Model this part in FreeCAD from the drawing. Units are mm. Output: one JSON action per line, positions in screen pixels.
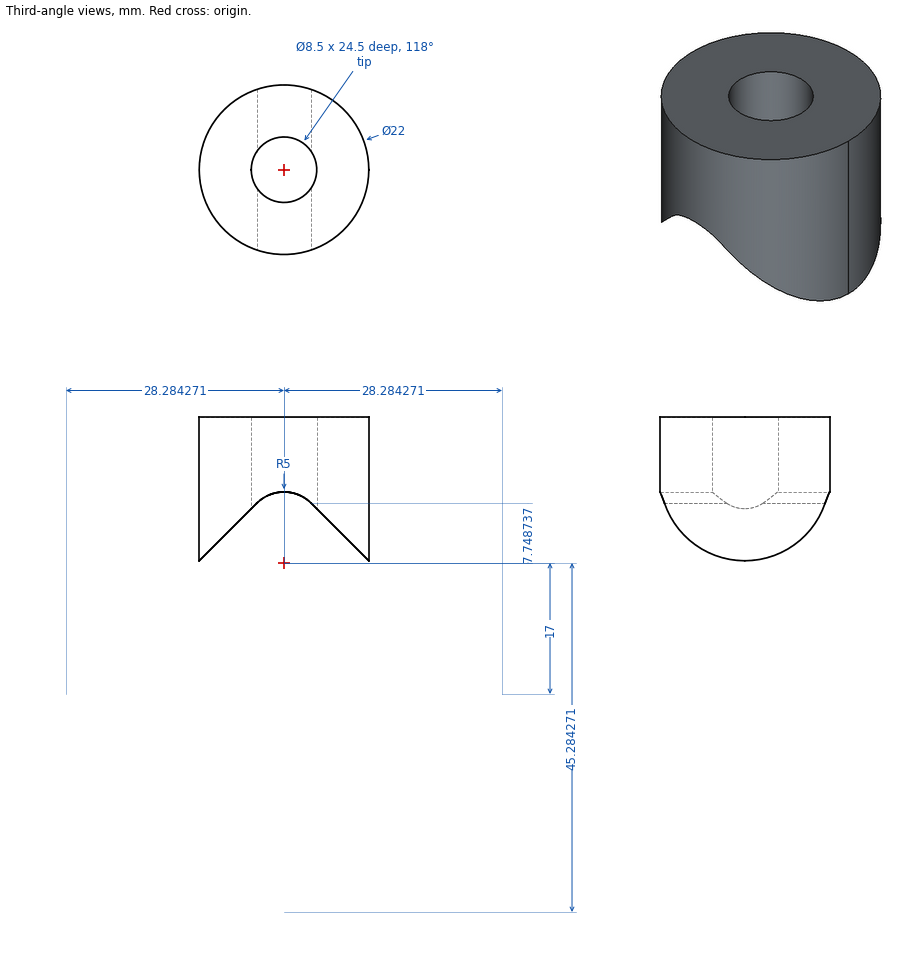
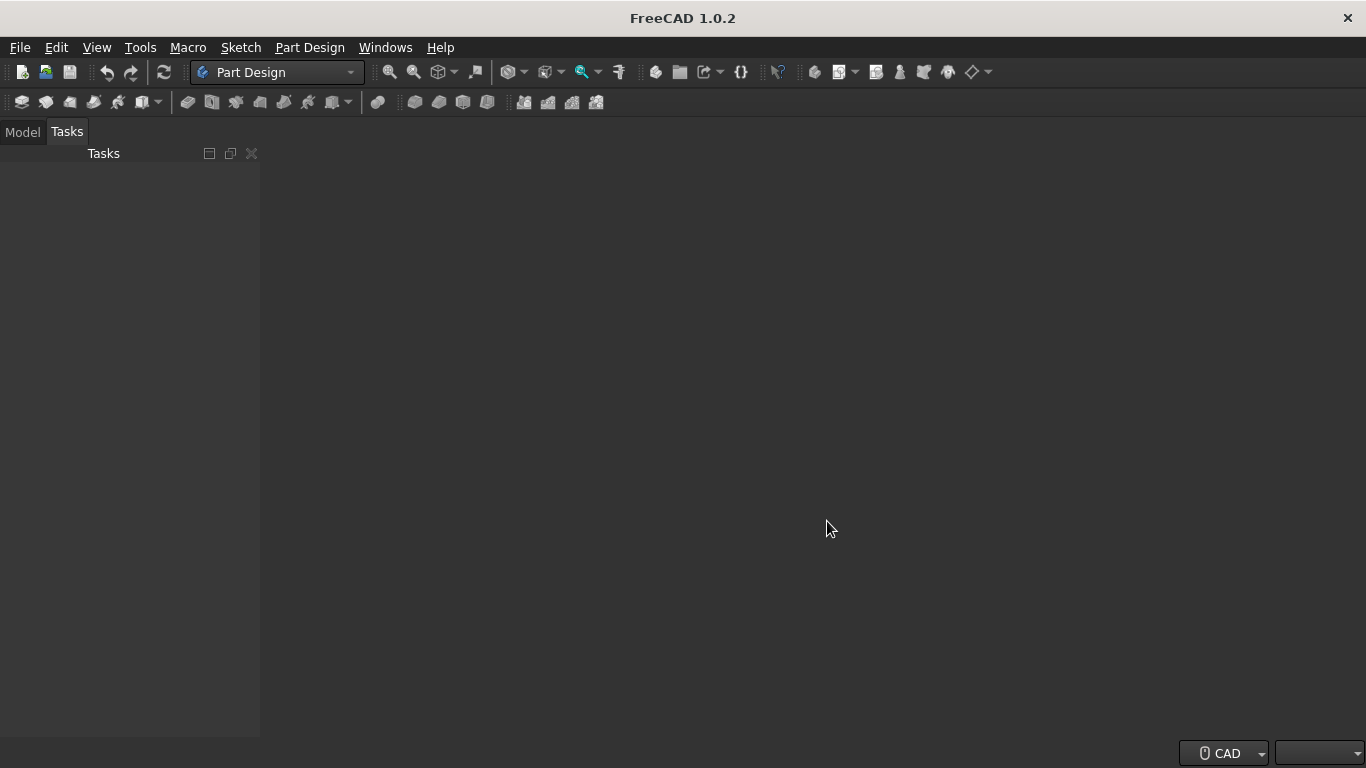
{"action": "key", "text": "ctrl+n"}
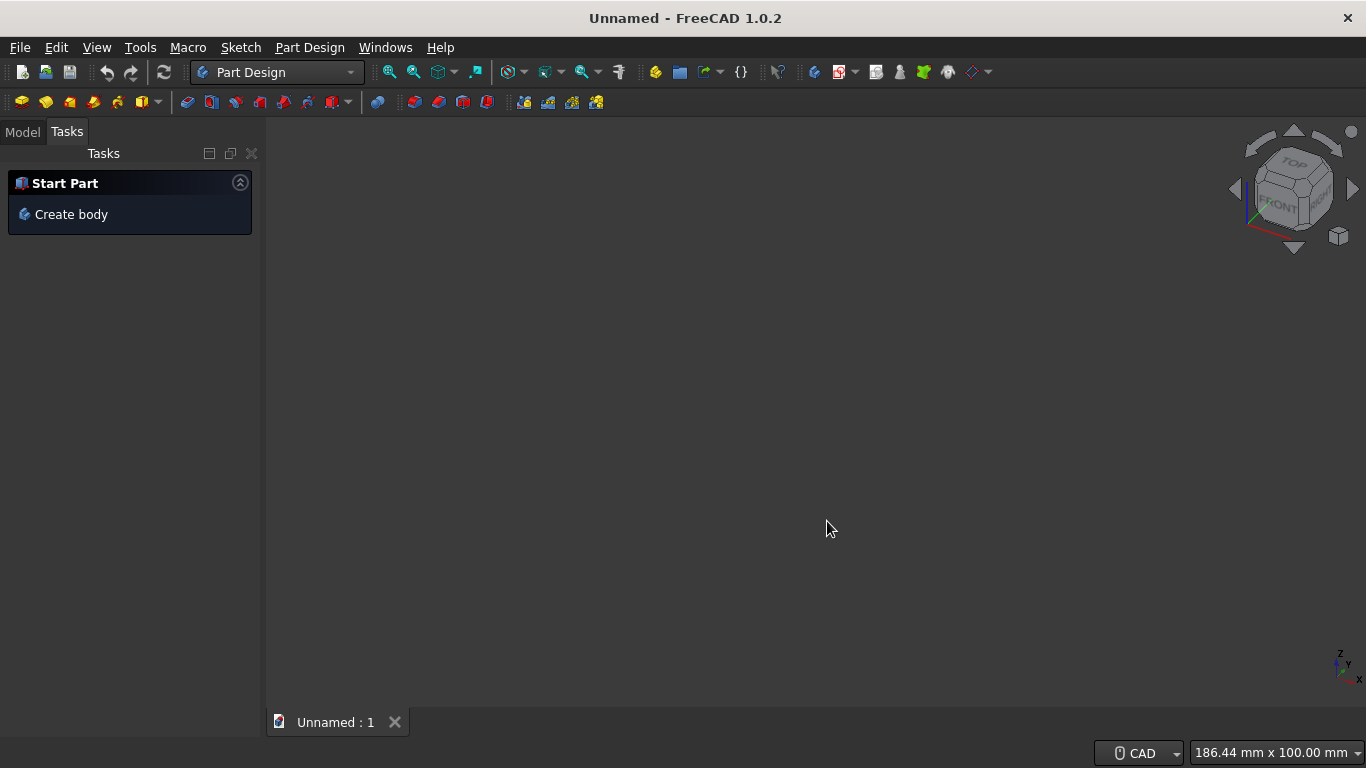
{"action": "left_click", "coordinate": [840, 72]}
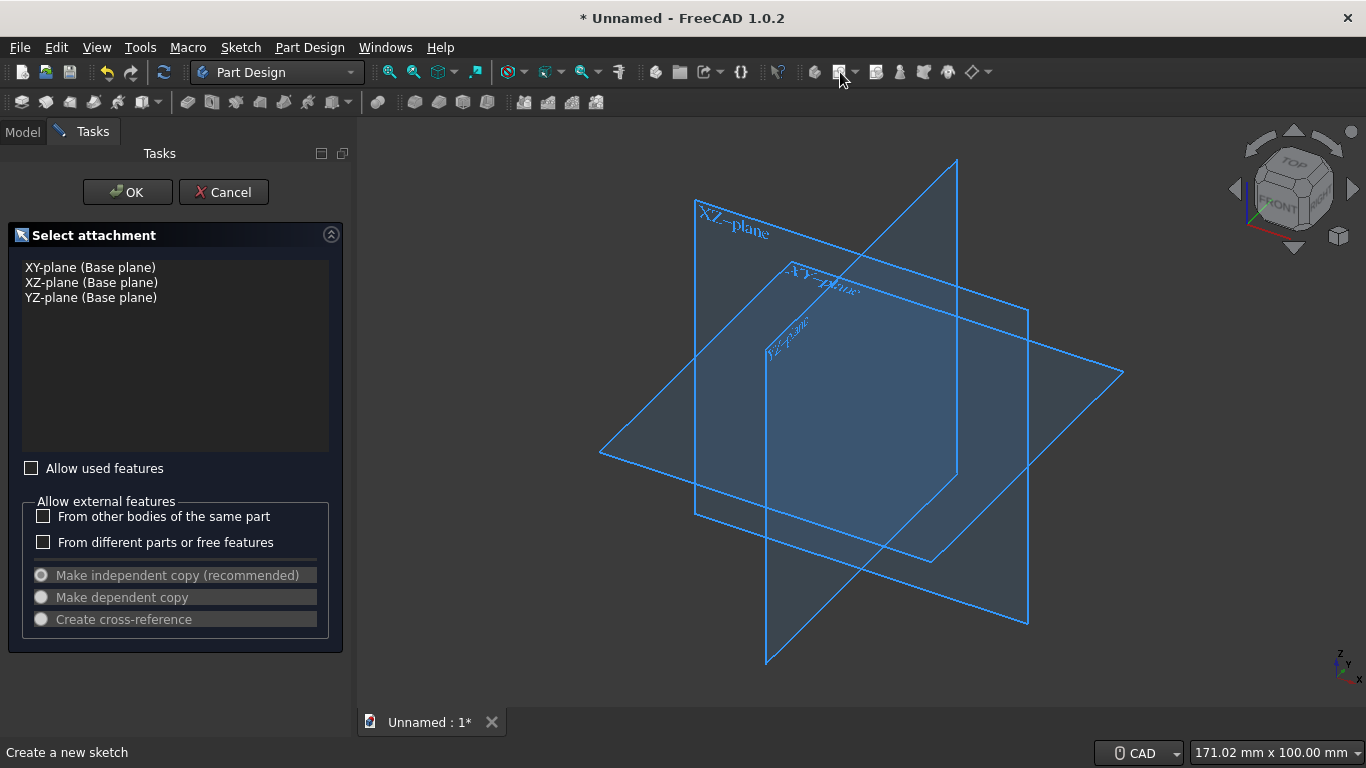
{"action": "left_click", "coordinate": [82, 268]}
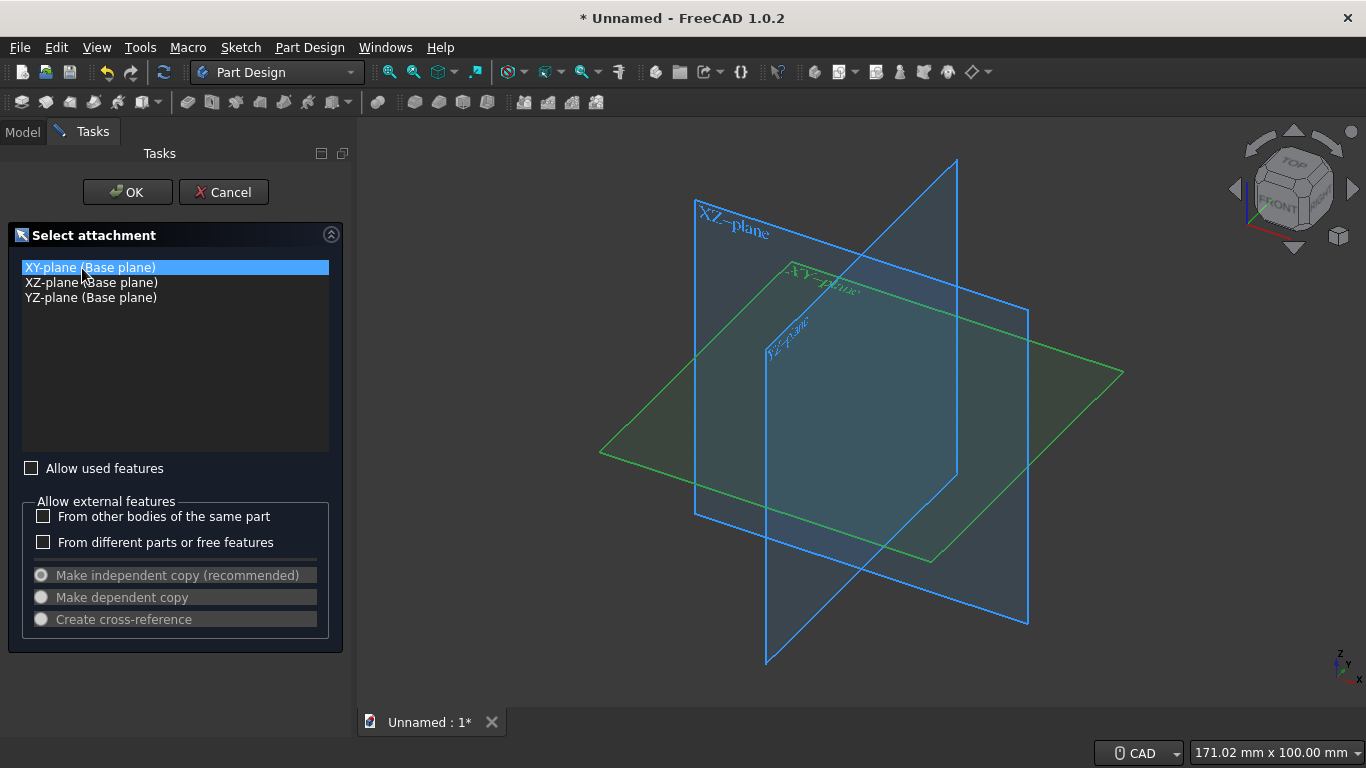
{"action": "left_click", "coordinate": [128, 192]}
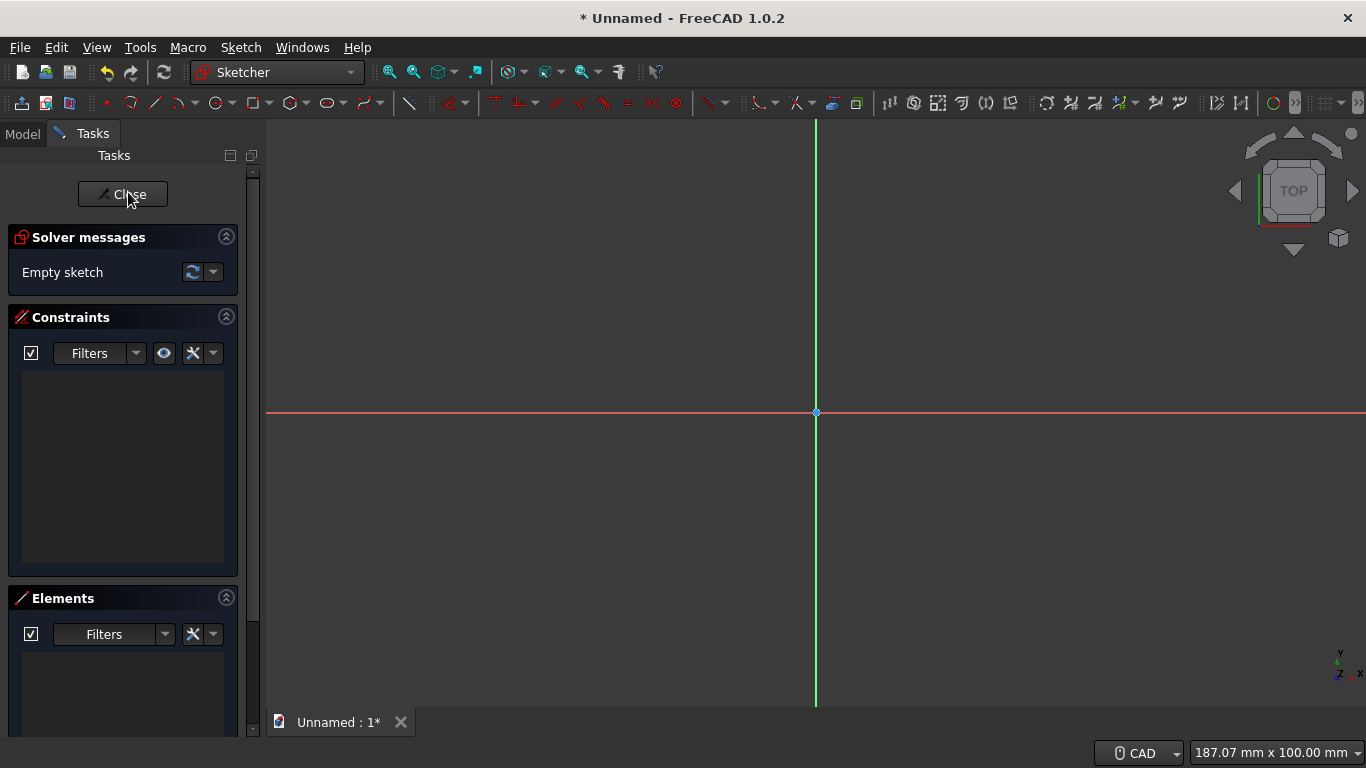
{"action": "scroll", "coordinate": [856, 413], "scroll_direction": "up", "scroll_amount": 5}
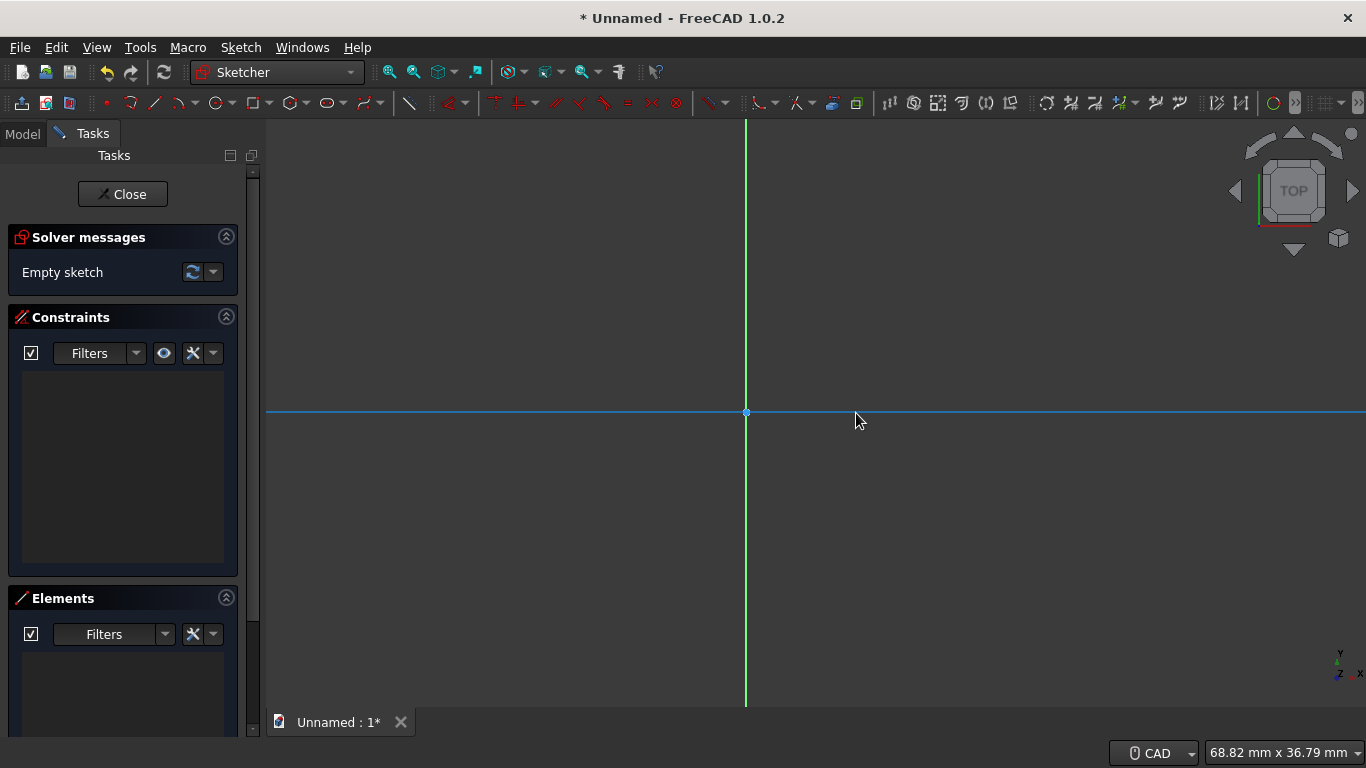
{"action": "key", "text": "g c"}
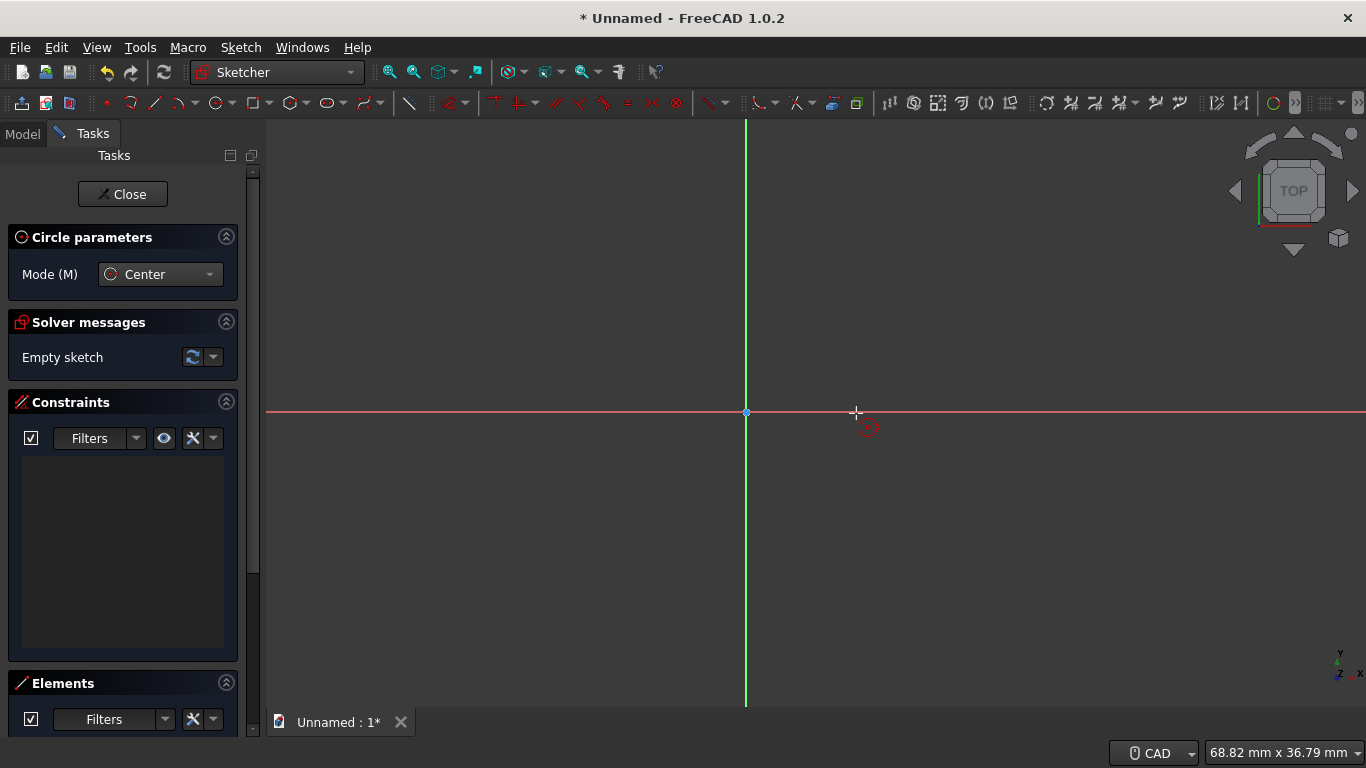
{"action": "left_click", "coordinate": [746, 412]}
{"action": "left_click", "coordinate": [871, 288]}
{"action": "key", "text": "Escape"}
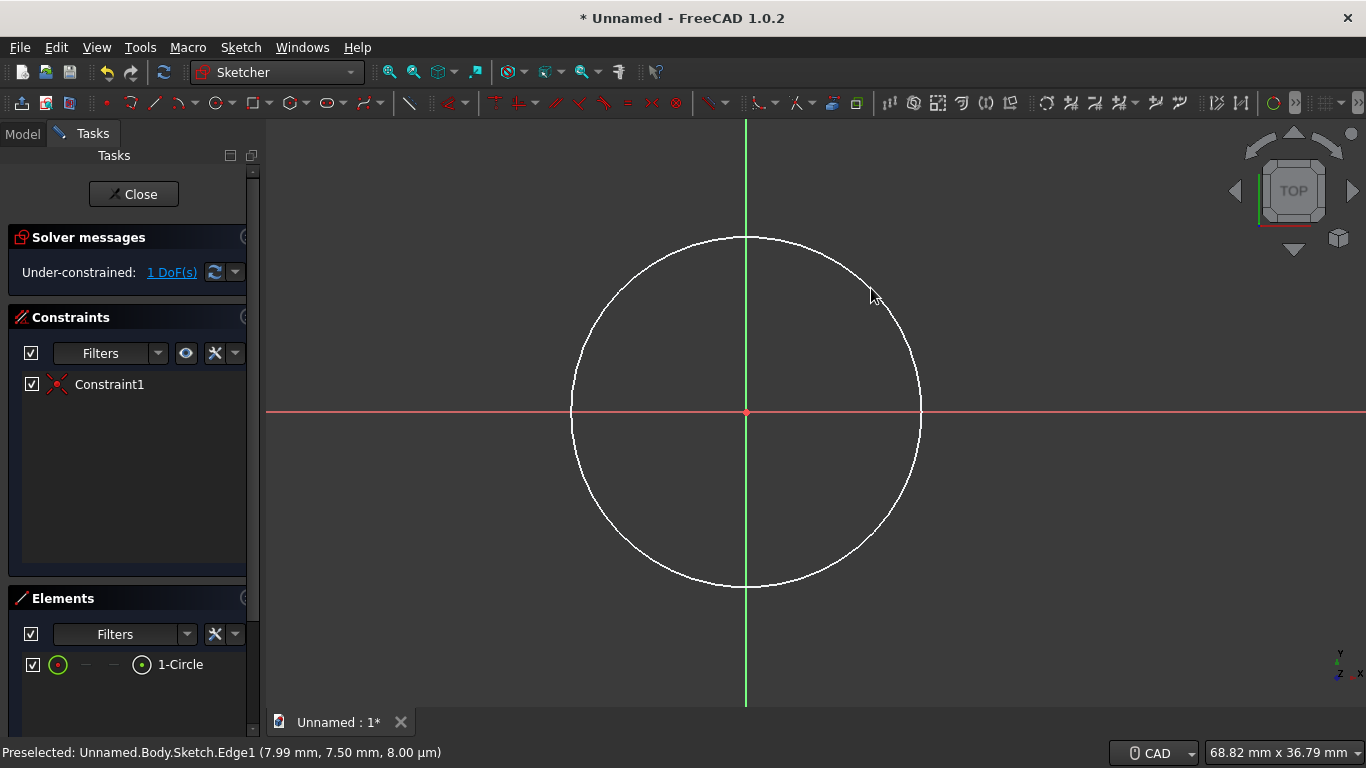
{"action": "key", "text": "d"}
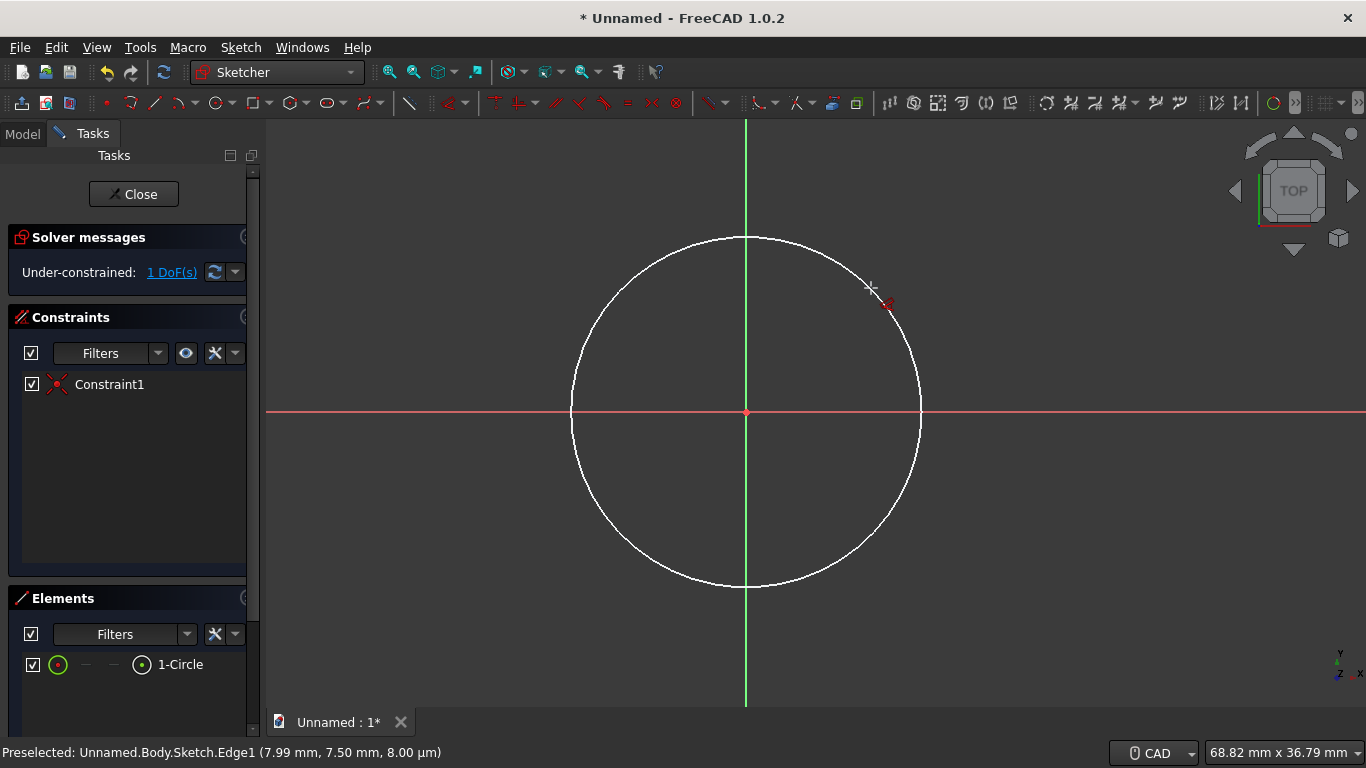
{"action": "left_click", "coordinate": [870, 288]}
{"action": "left_click", "coordinate": [893, 265]}